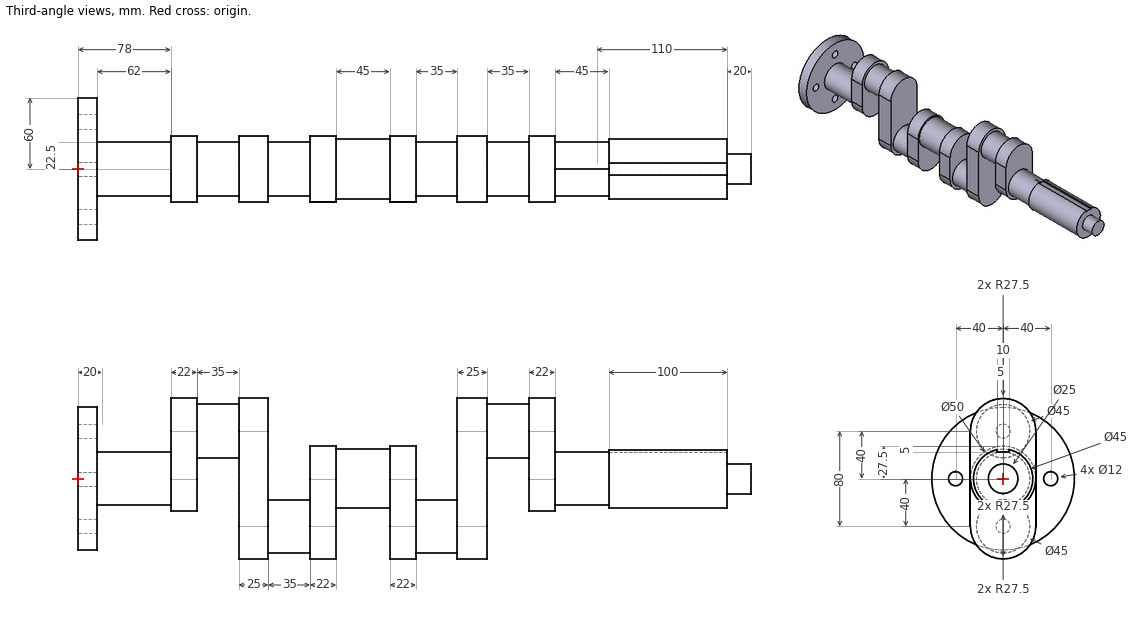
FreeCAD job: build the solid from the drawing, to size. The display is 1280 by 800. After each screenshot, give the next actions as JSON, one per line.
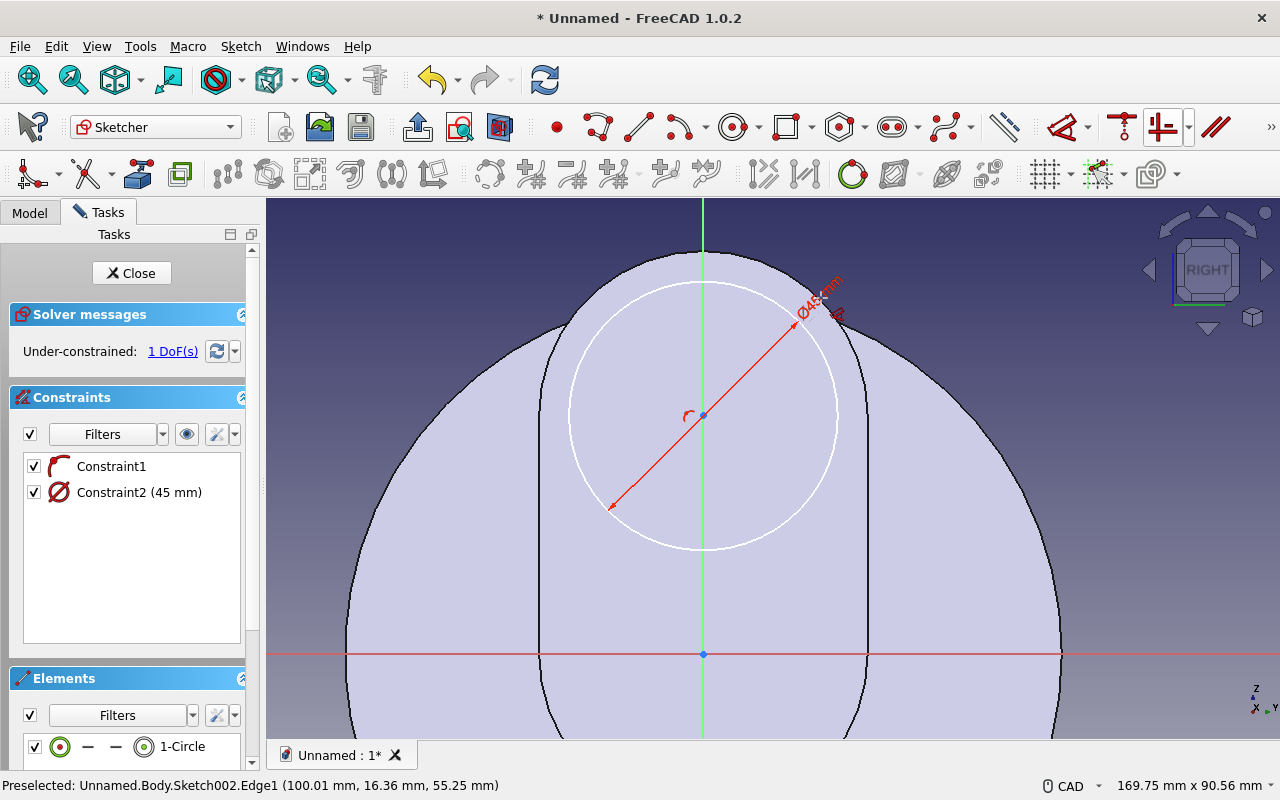
{"action": "left_click", "coordinate": [703, 416]}
{"action": "left_click", "coordinate": [737, 480]}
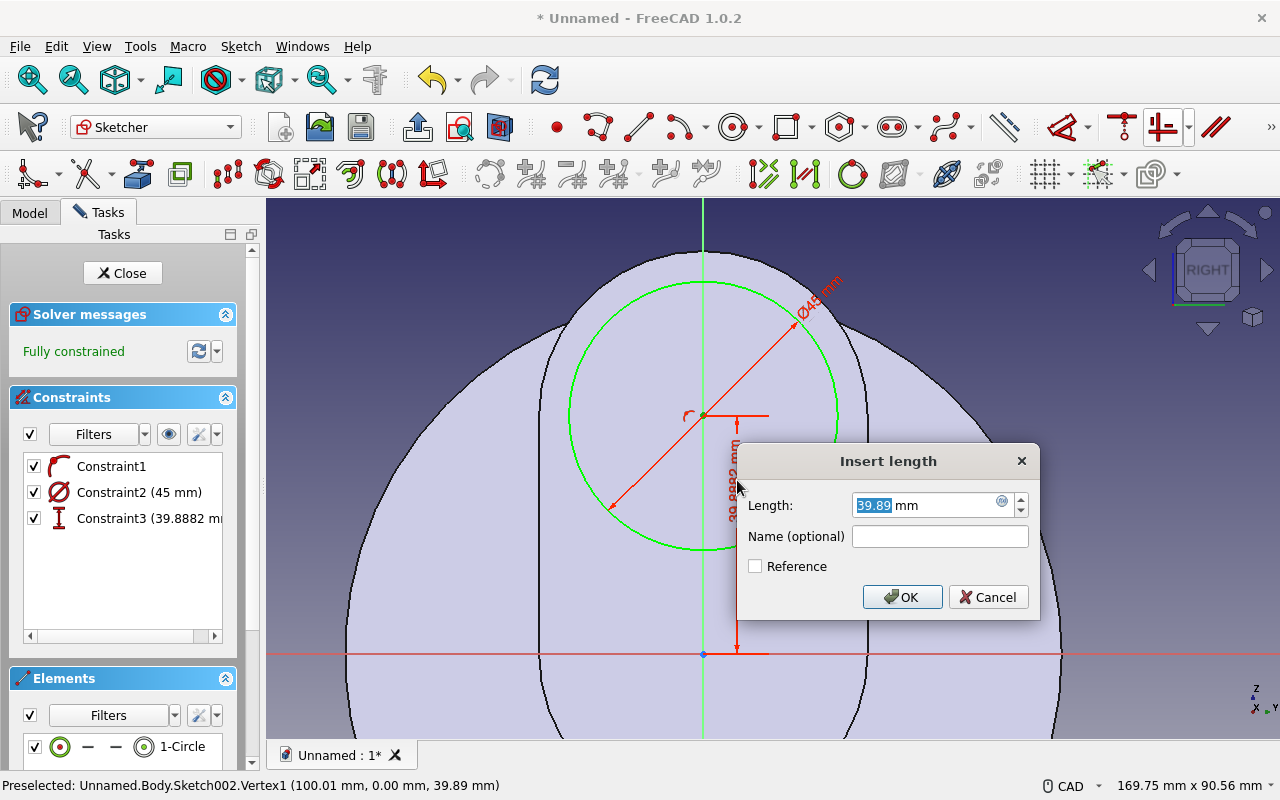
{"action": "type", "text": "40"}
{"action": "key", "text": "Return"}
{"action": "key", "text": "Escape"}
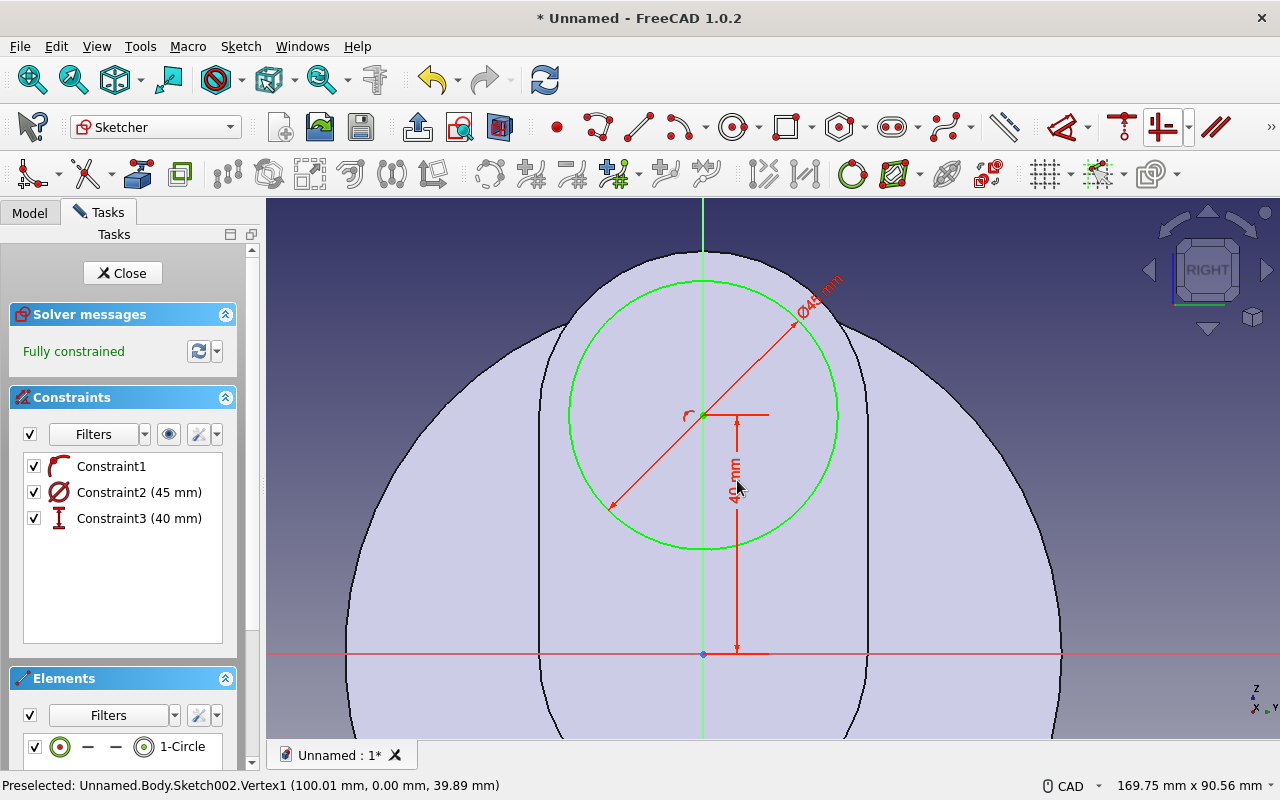
{"action": "left_click", "coordinate": [123, 273]}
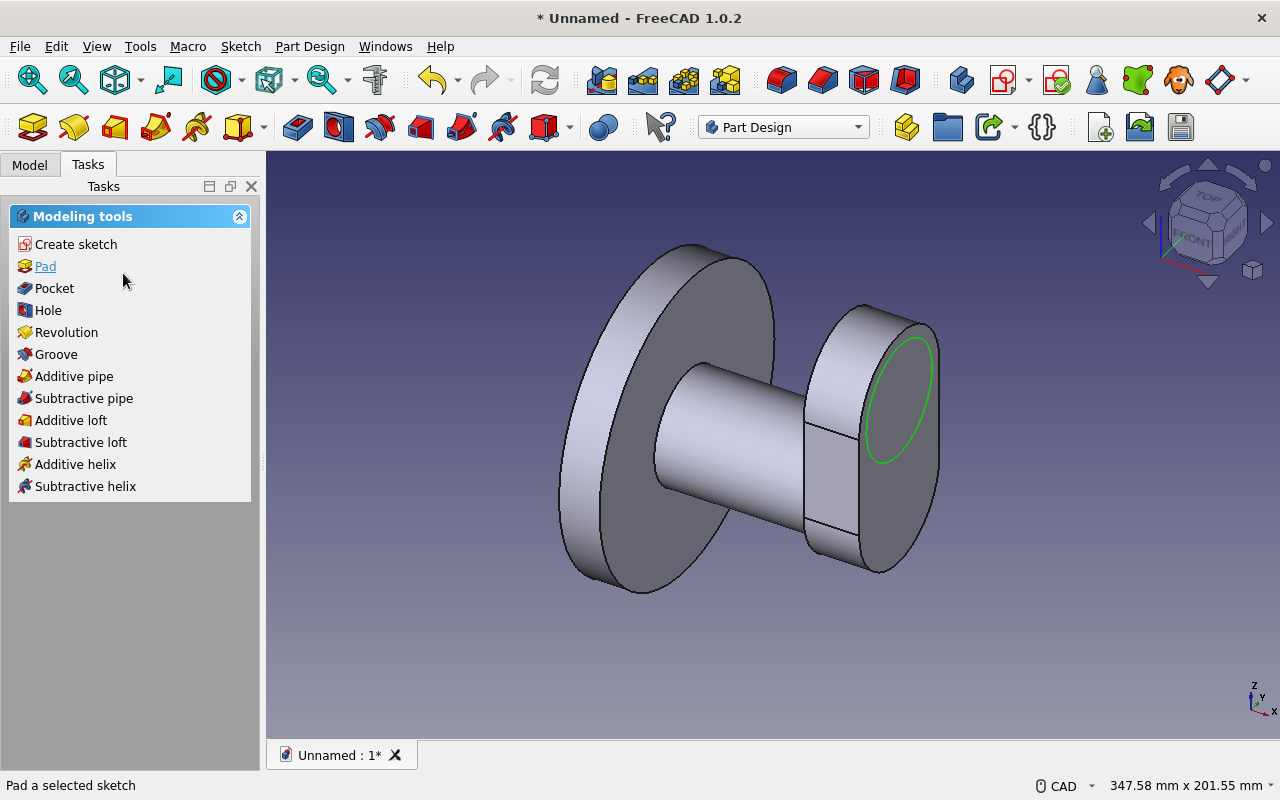
{"action": "left_click", "coordinate": [33, 128]}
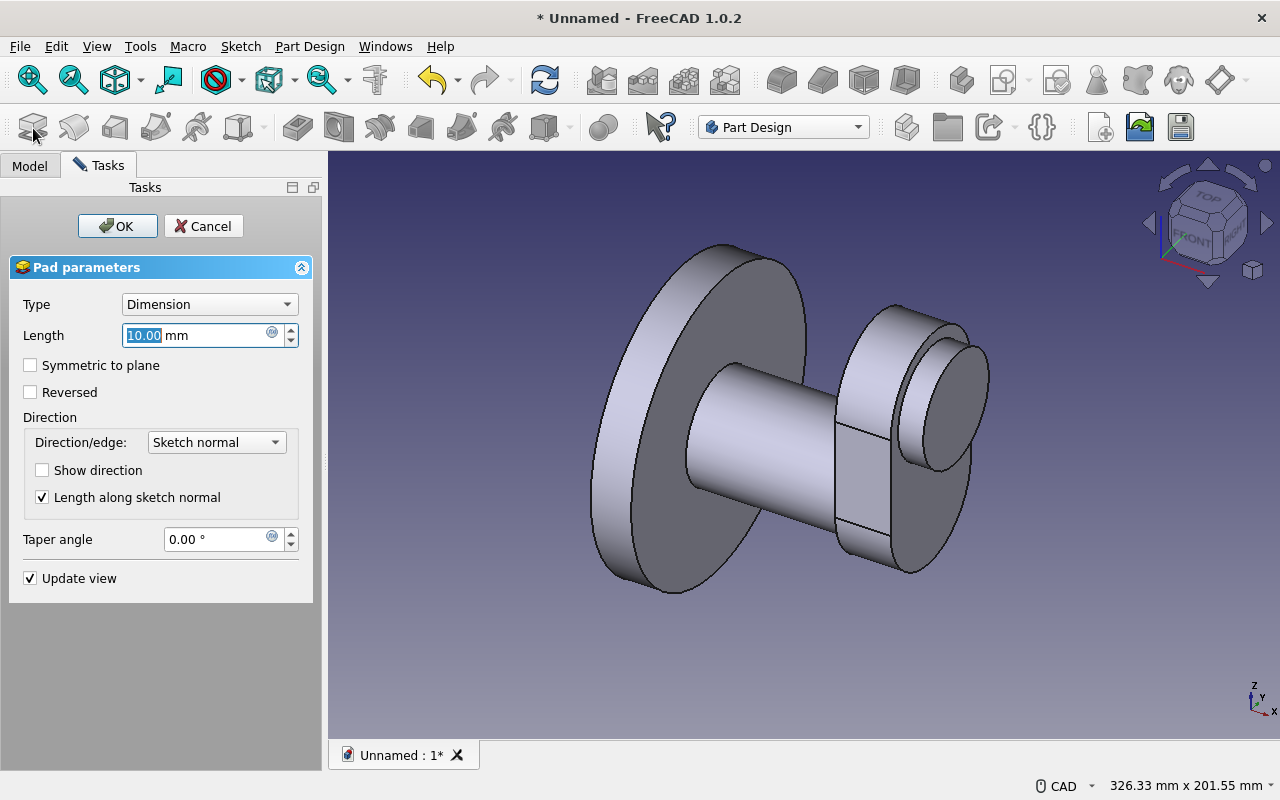
{"action": "type", "text": "35"}
{"action": "key", "text": "Tab"}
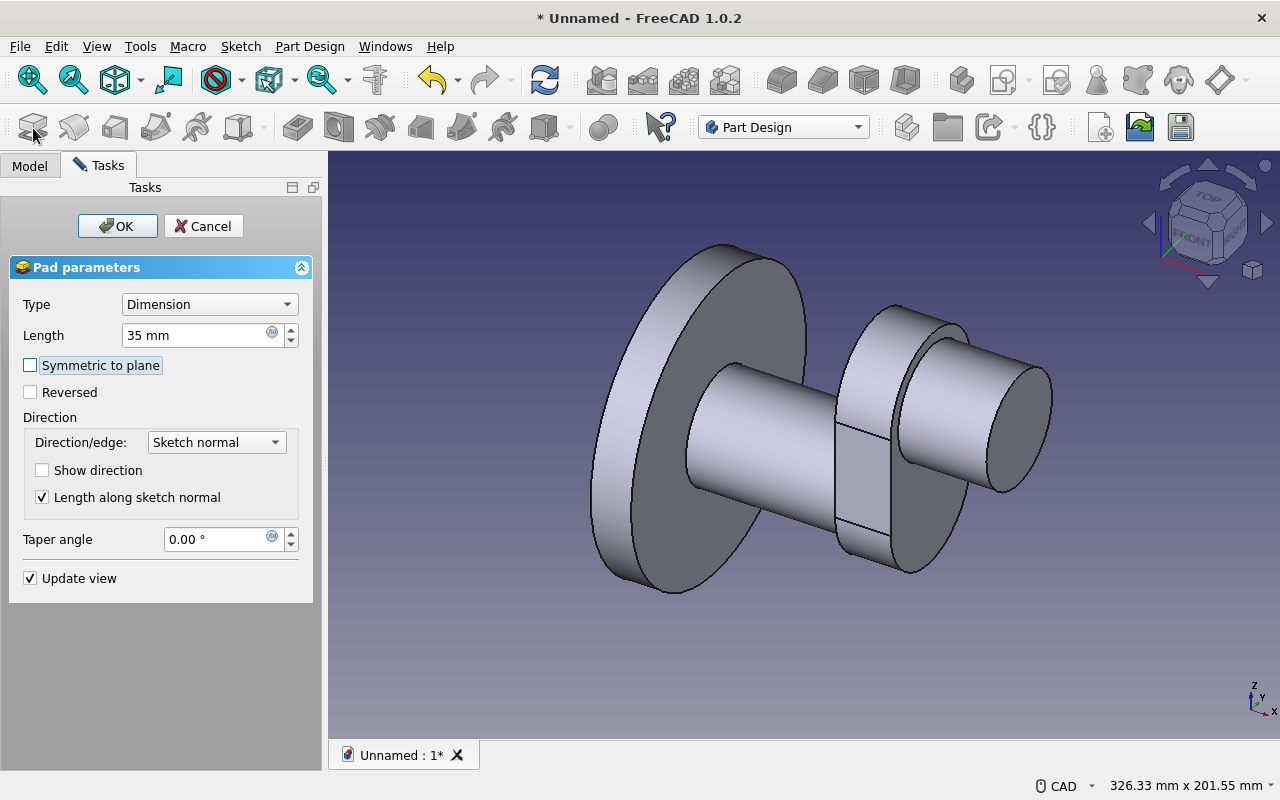
{"action": "left_click", "coordinate": [118, 226]}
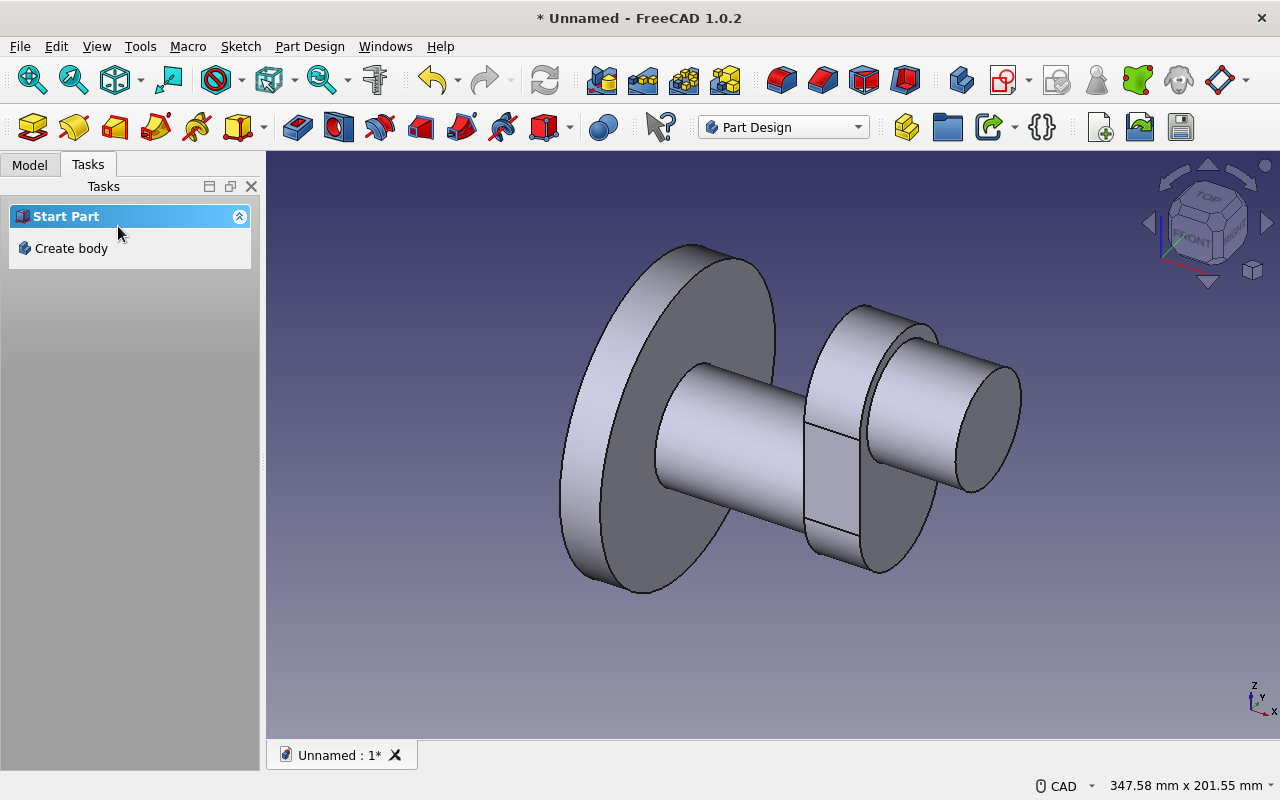
{"action": "left_click", "coordinate": [33, 80]}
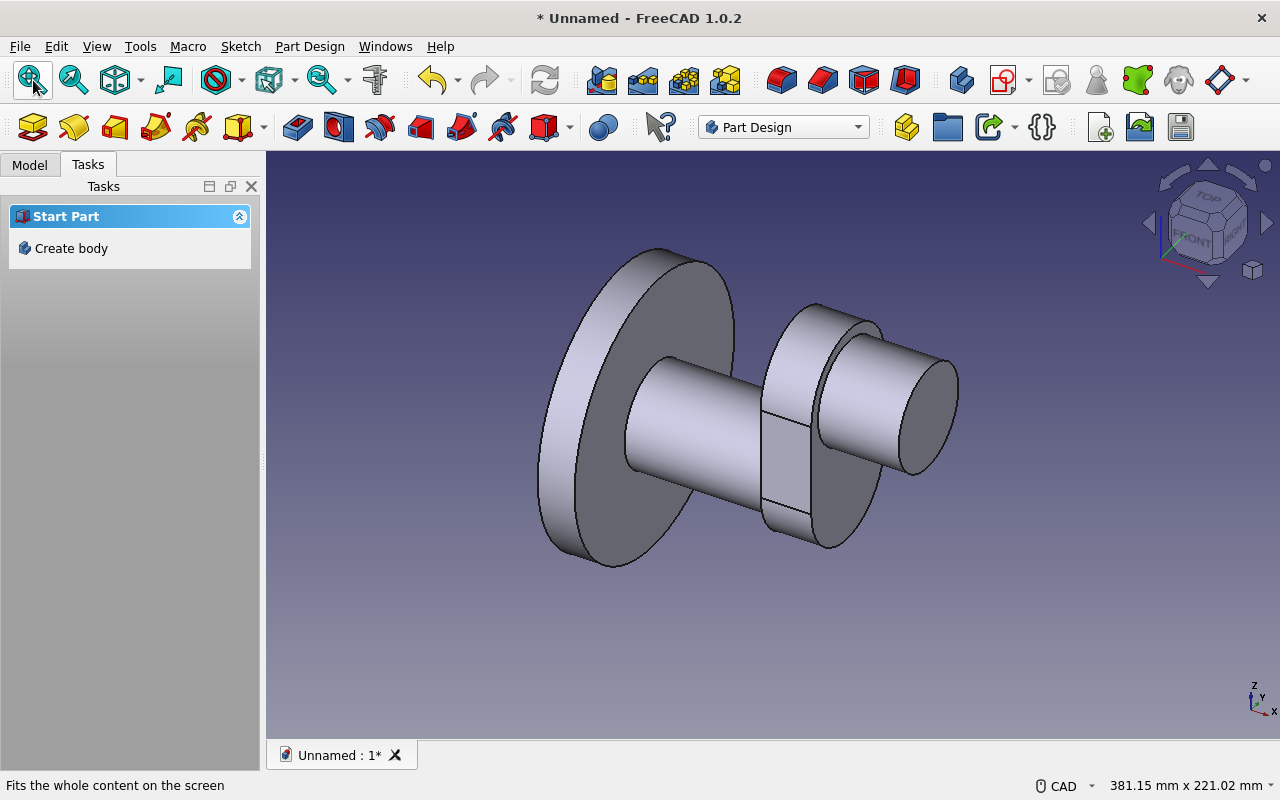
{"action": "left_click", "coordinate": [929, 417]}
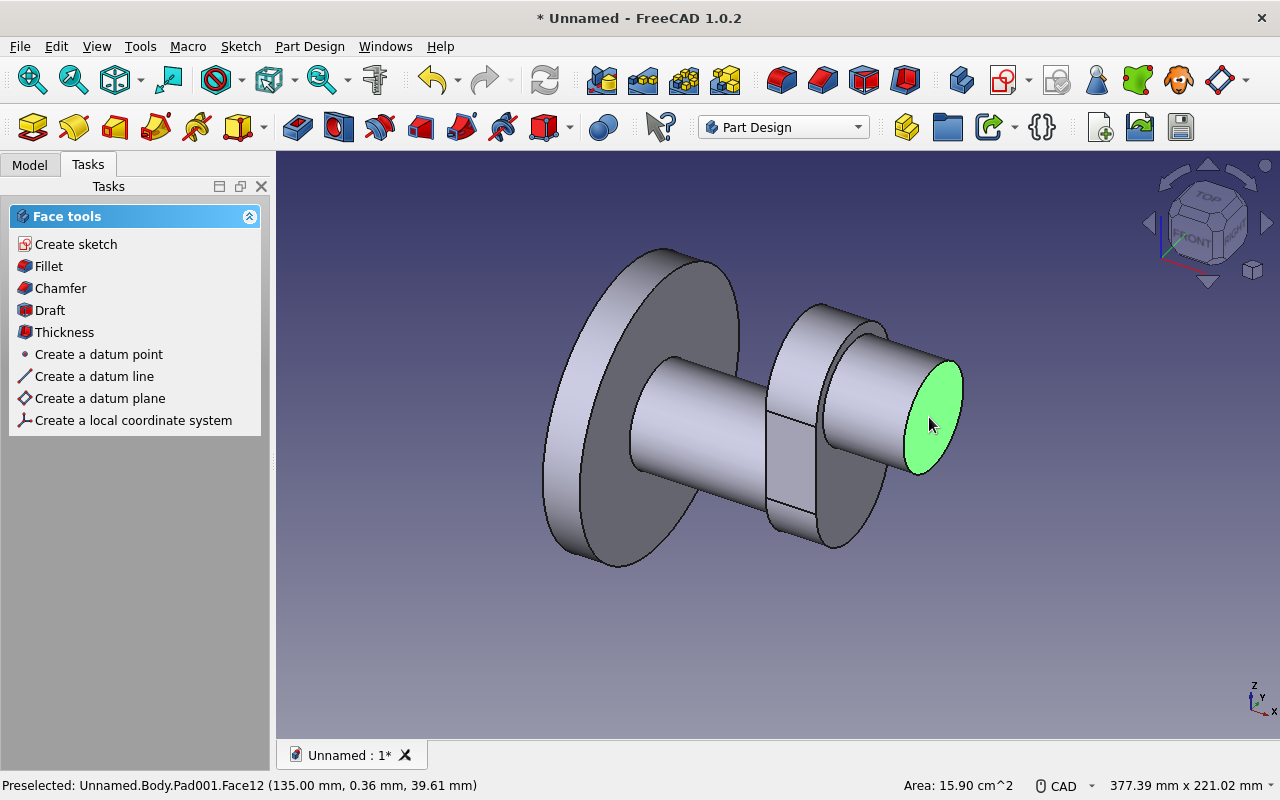
{"action": "left_click", "coordinate": [1002, 80]}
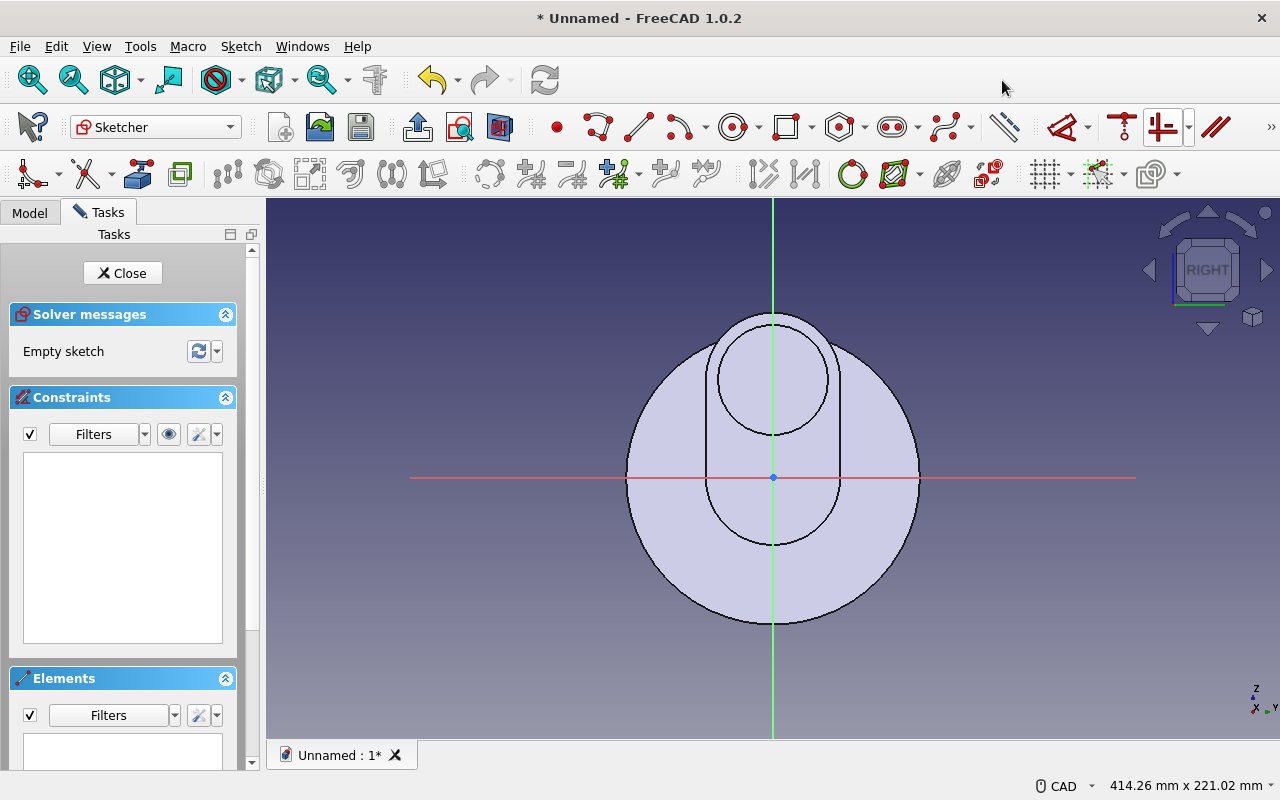
{"action": "left_click", "coordinate": [892, 128]}